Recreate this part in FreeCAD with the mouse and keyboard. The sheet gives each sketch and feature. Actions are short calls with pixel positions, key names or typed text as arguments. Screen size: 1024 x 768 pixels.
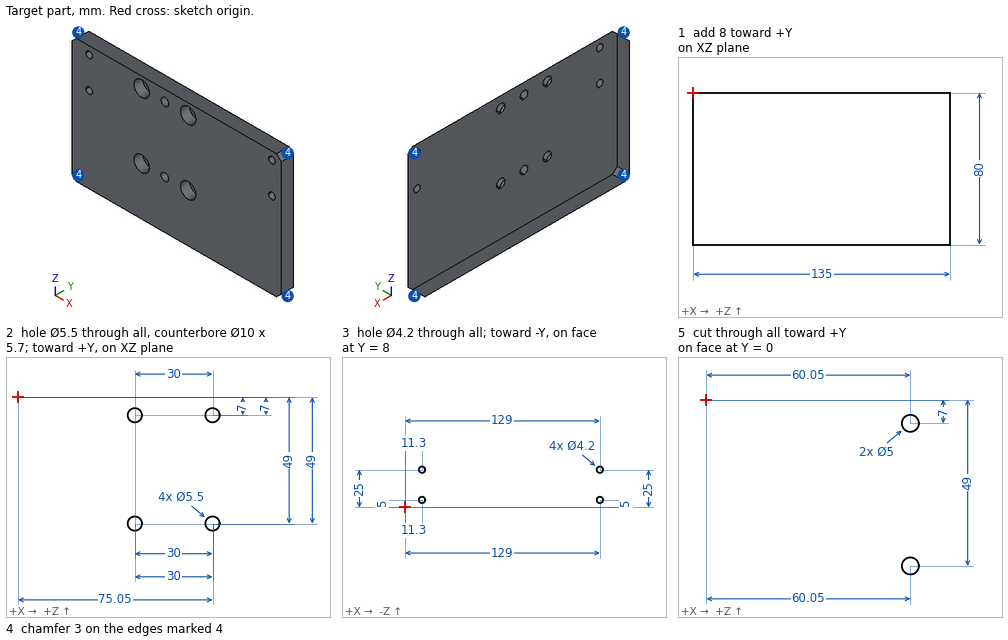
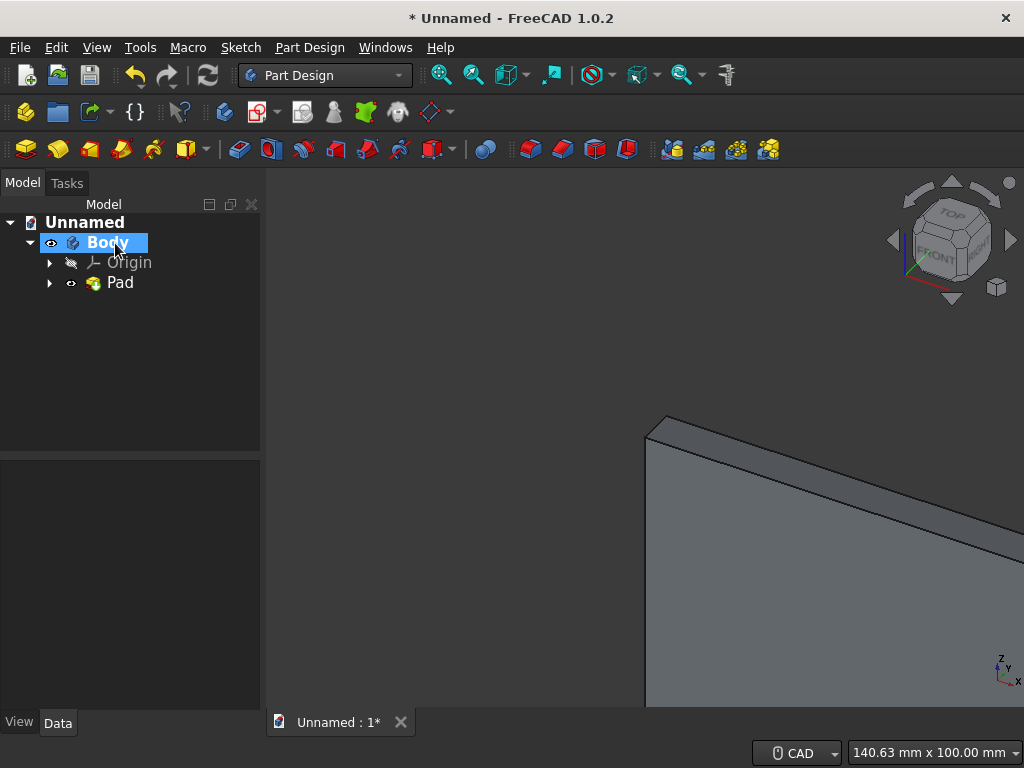
key(v)
key(f)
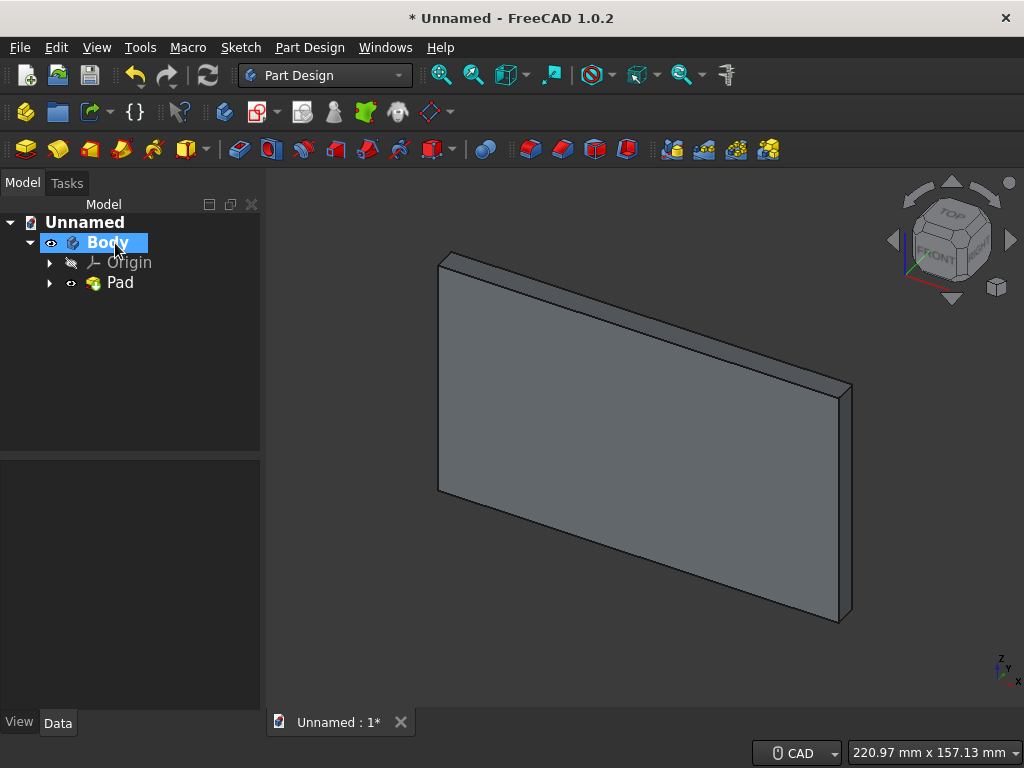
click(258, 112)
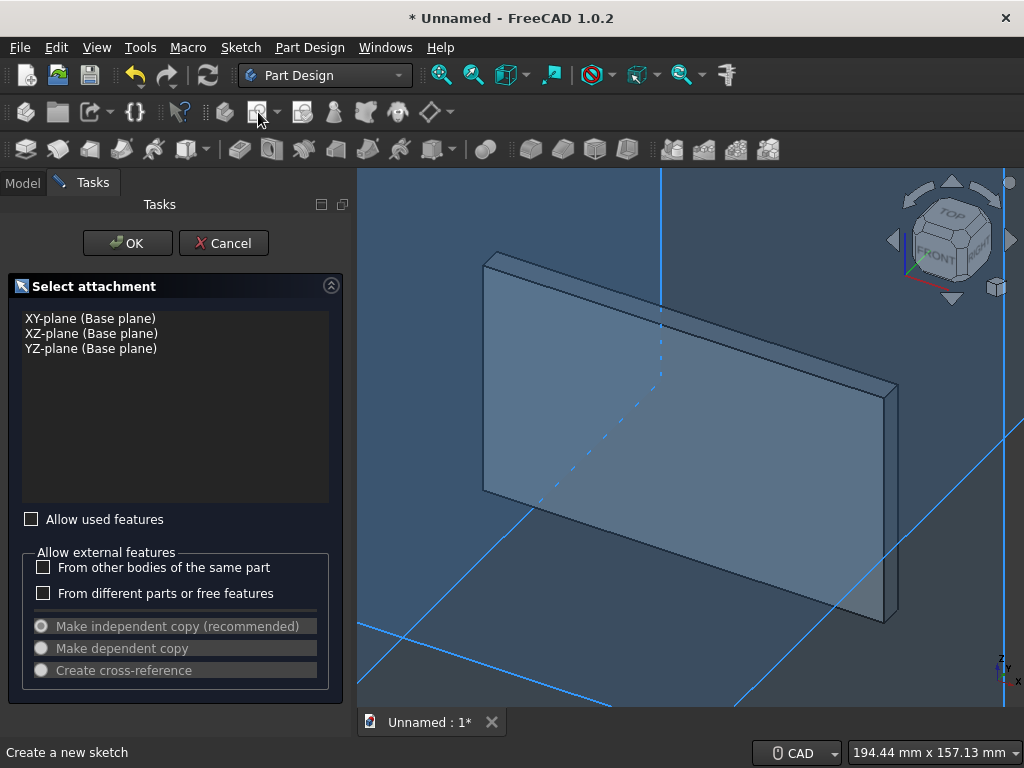
click(82, 334)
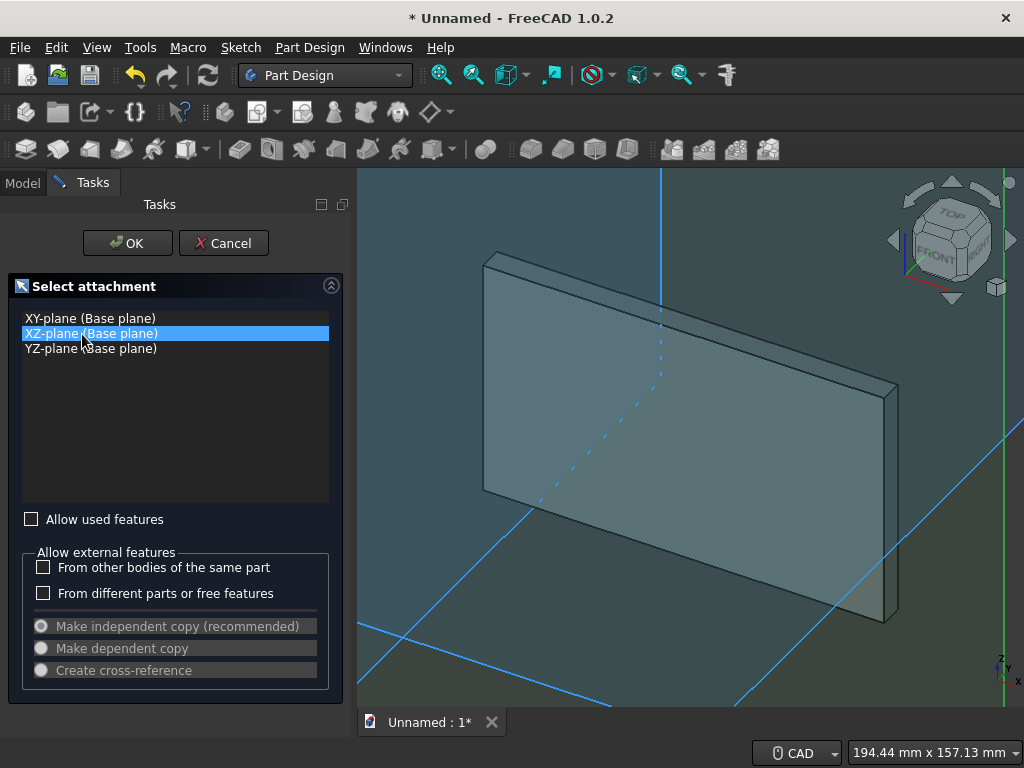
click(128, 243)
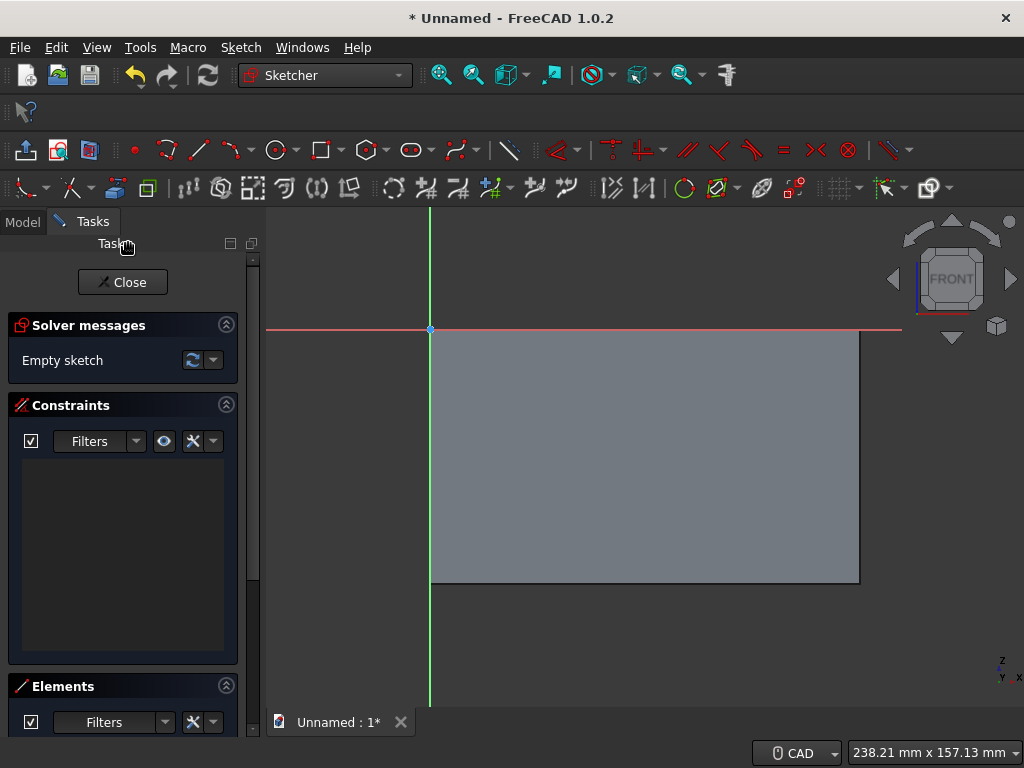
scroll(508, 321, up, 2)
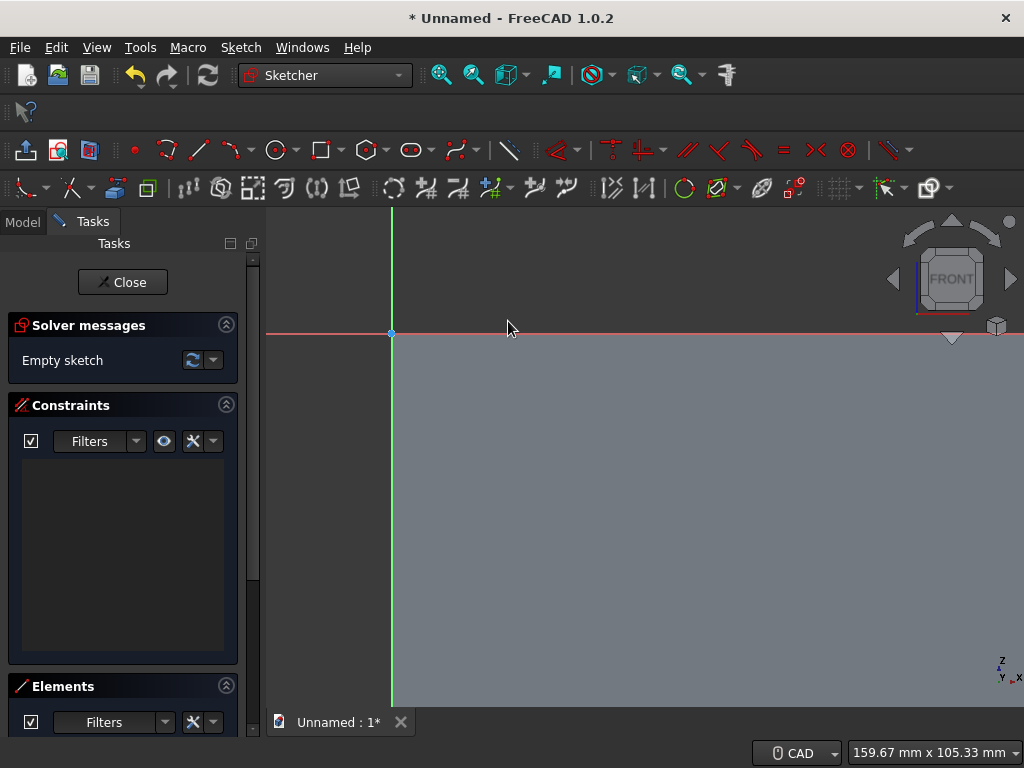
key(g)
key(c)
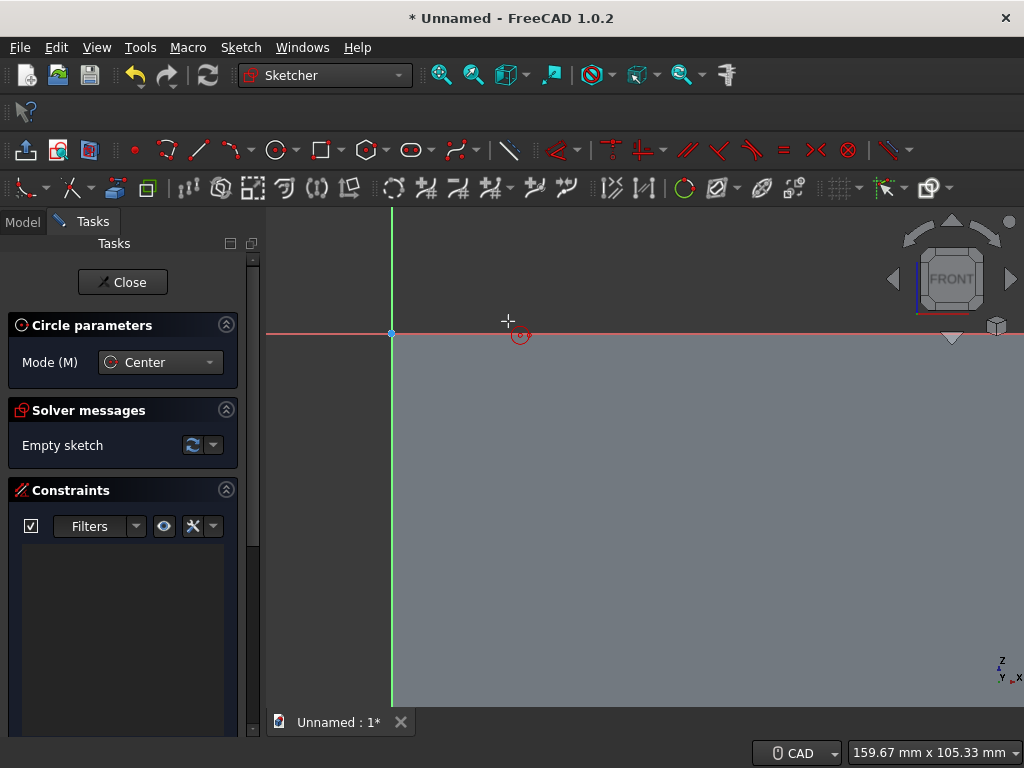
scroll(748, 567, up, 3)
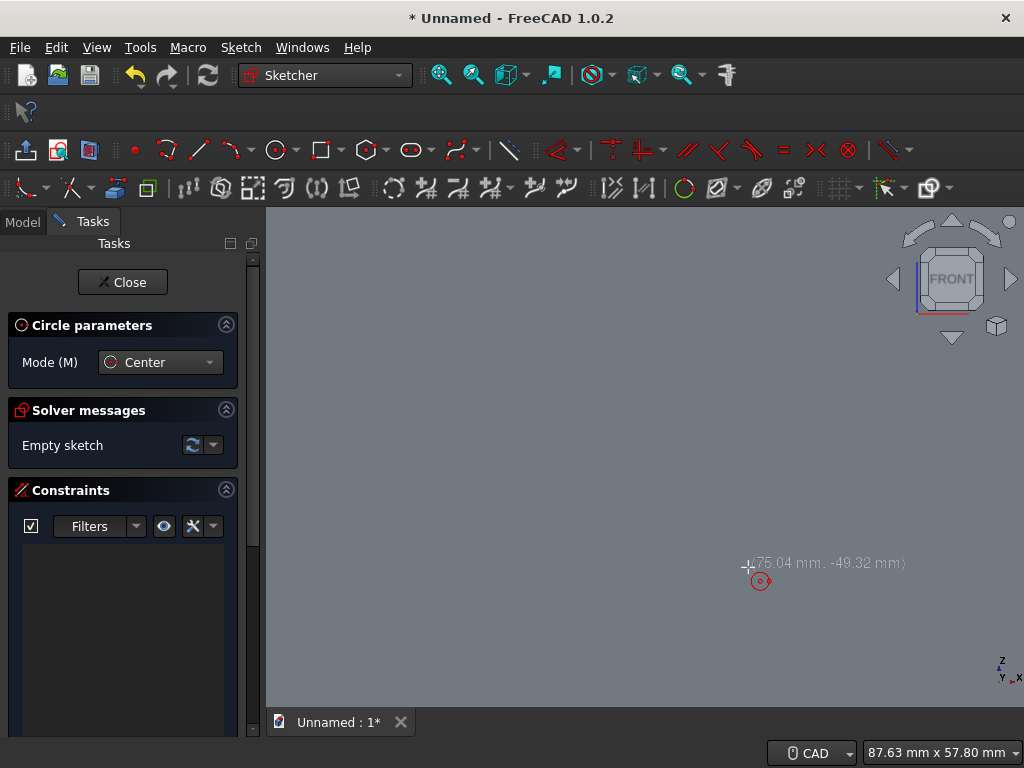
click(748, 565)
move(764, 549)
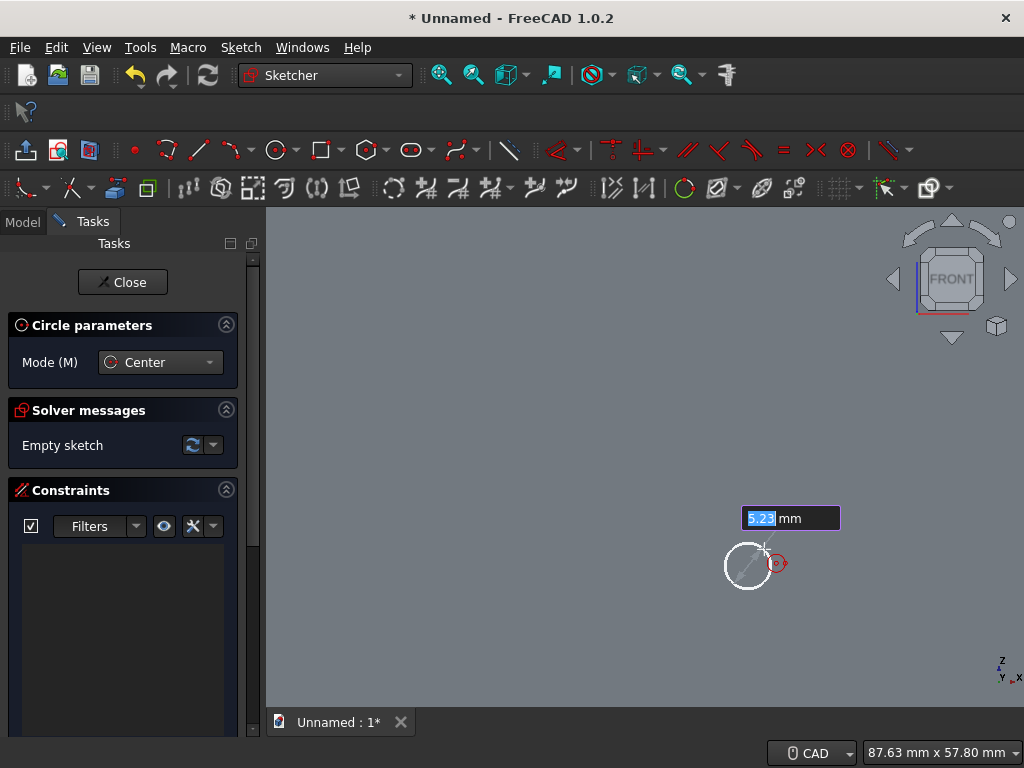
text(5.5)
key(Return)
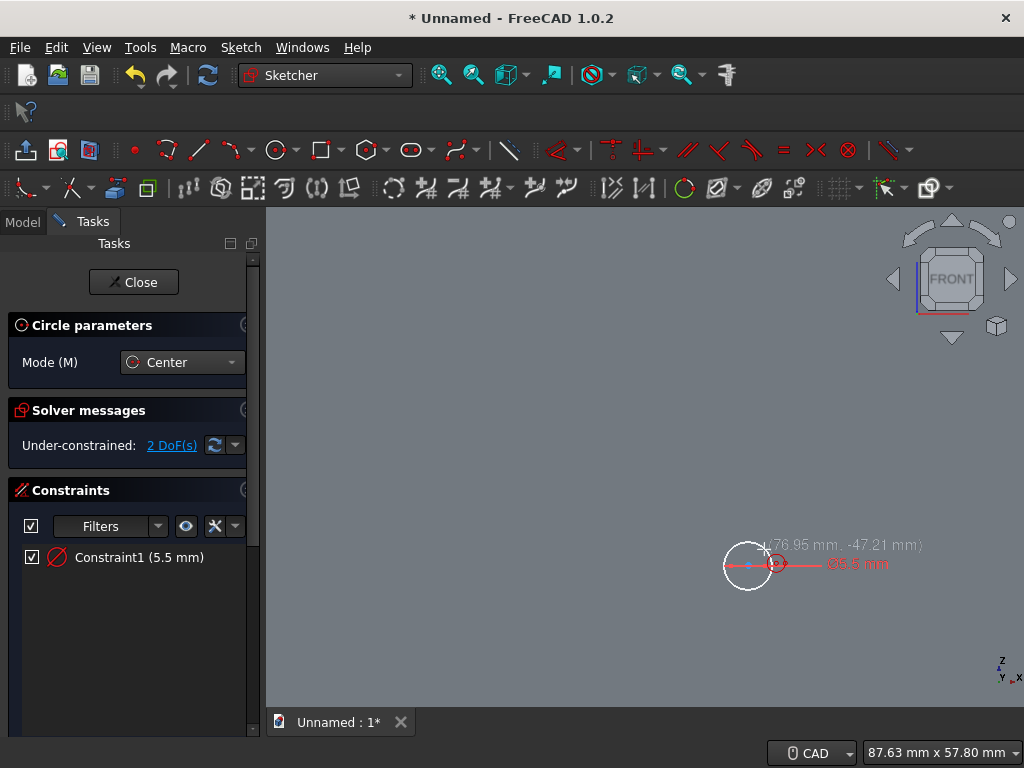
click(488, 565)
move(505, 549)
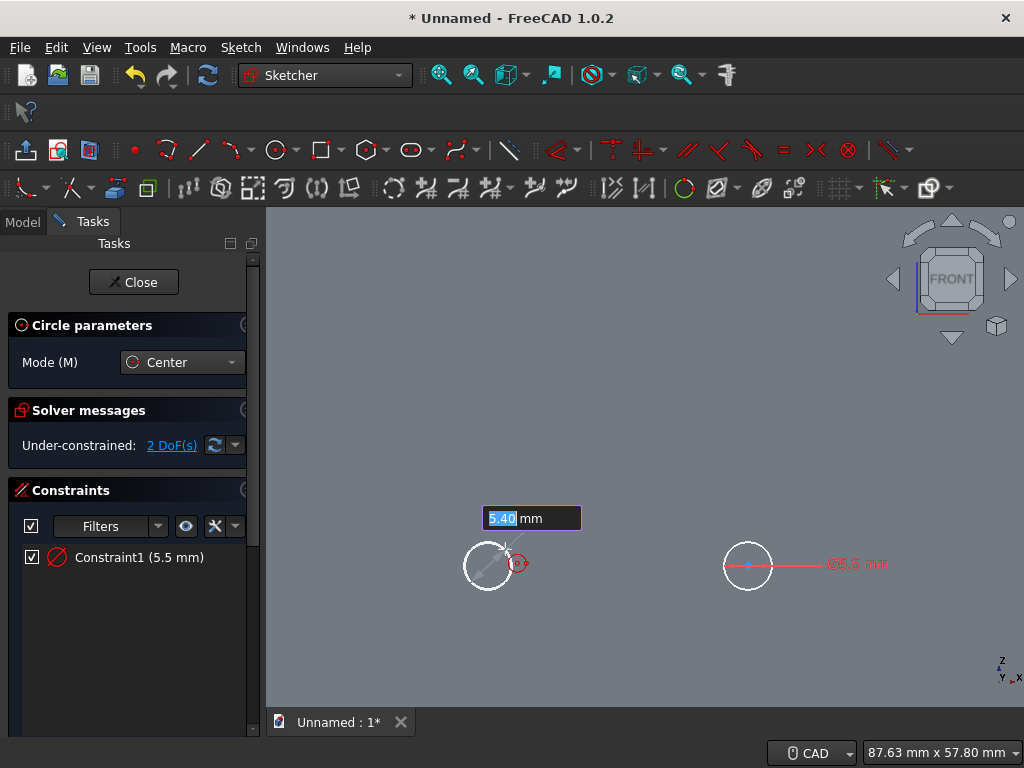
text(5.5)
key(Return)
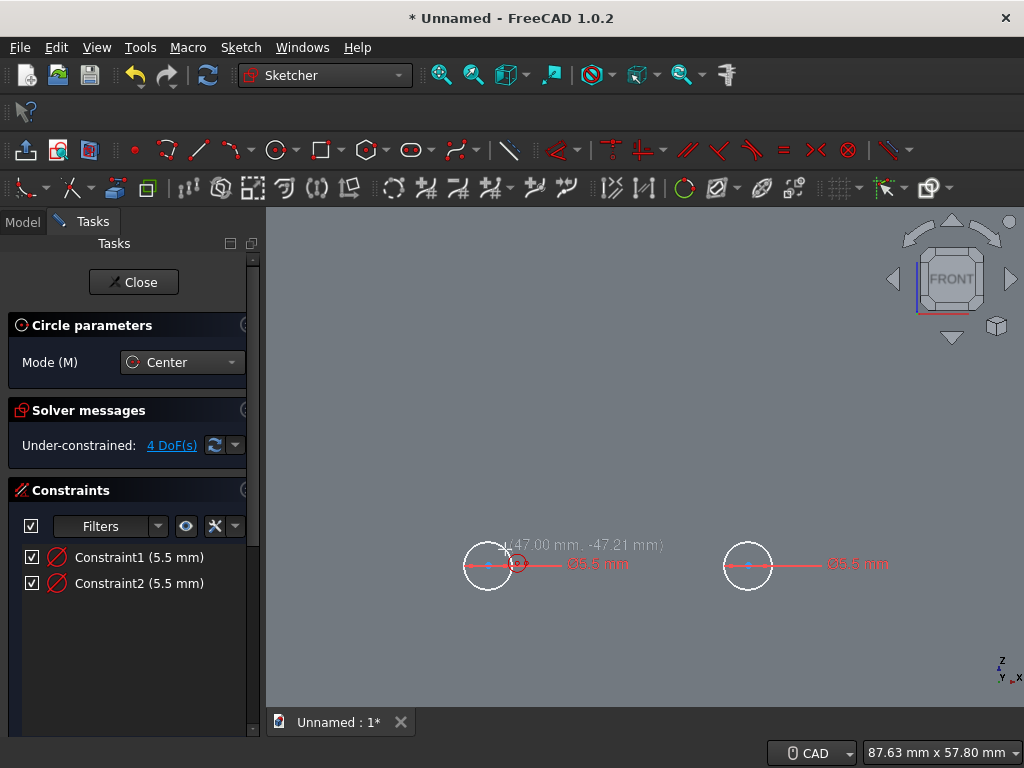
scroll(749, 568, down, 3)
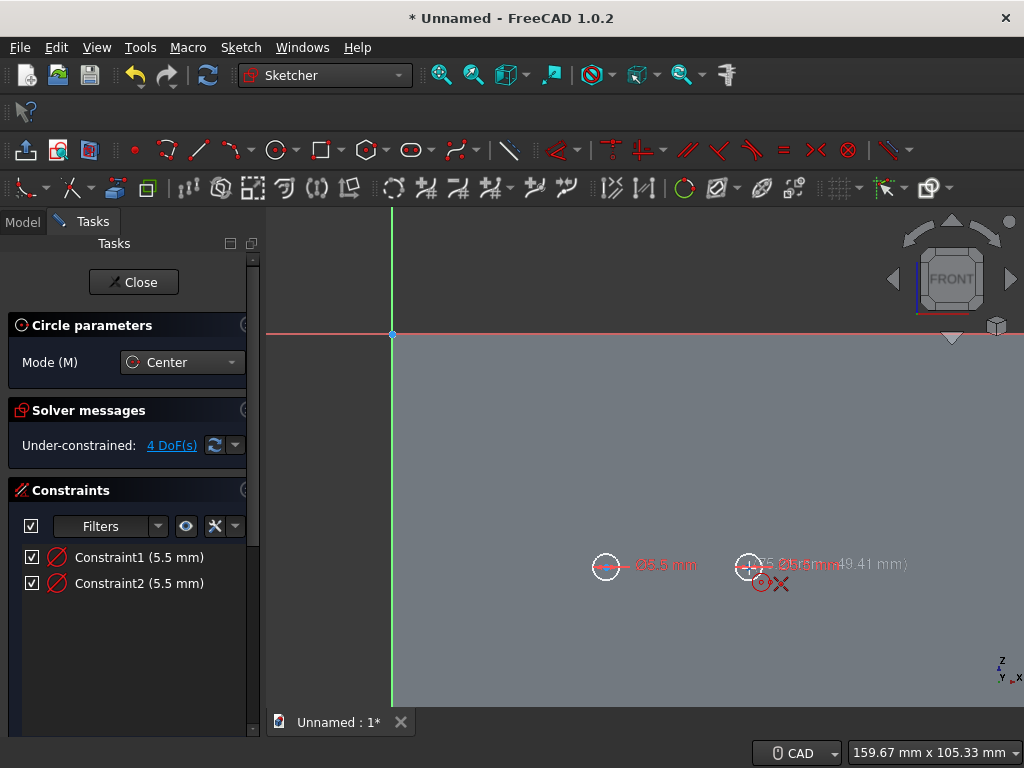
scroll(606, 368, up, 3)